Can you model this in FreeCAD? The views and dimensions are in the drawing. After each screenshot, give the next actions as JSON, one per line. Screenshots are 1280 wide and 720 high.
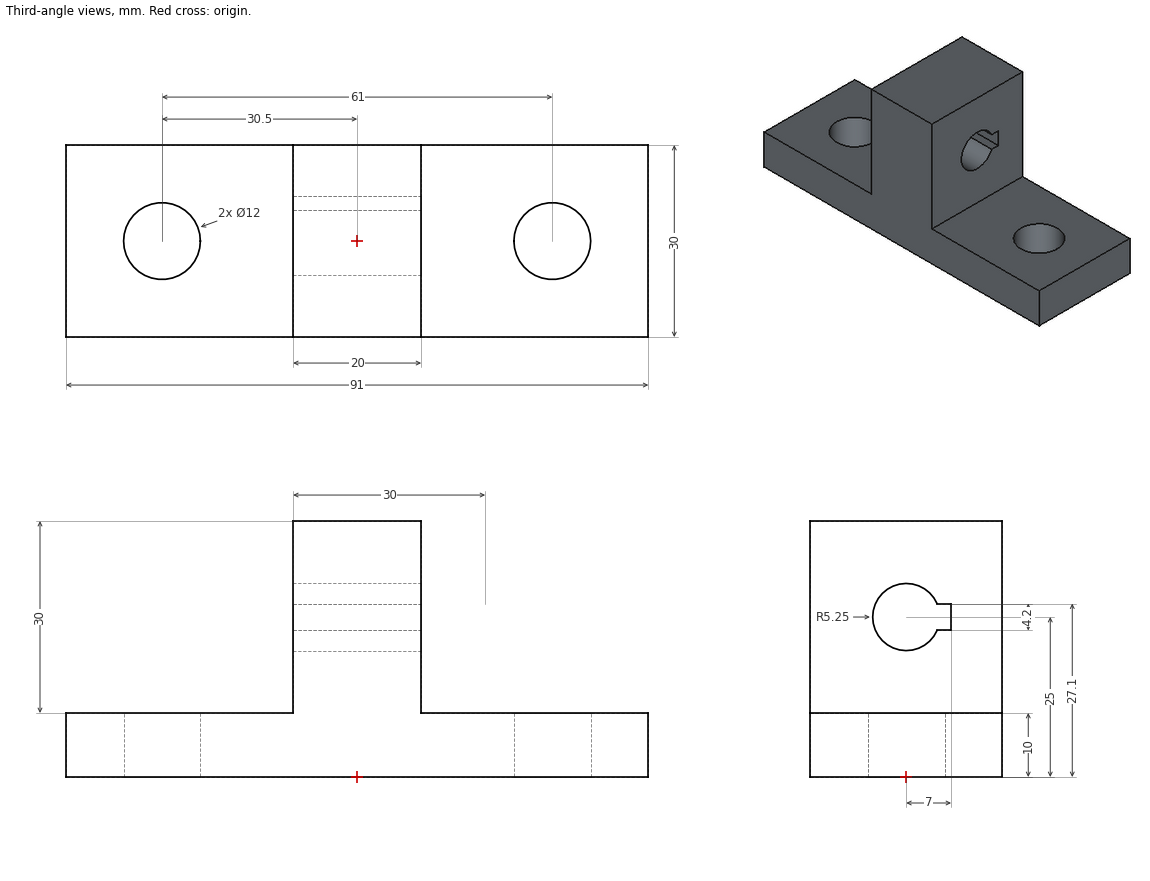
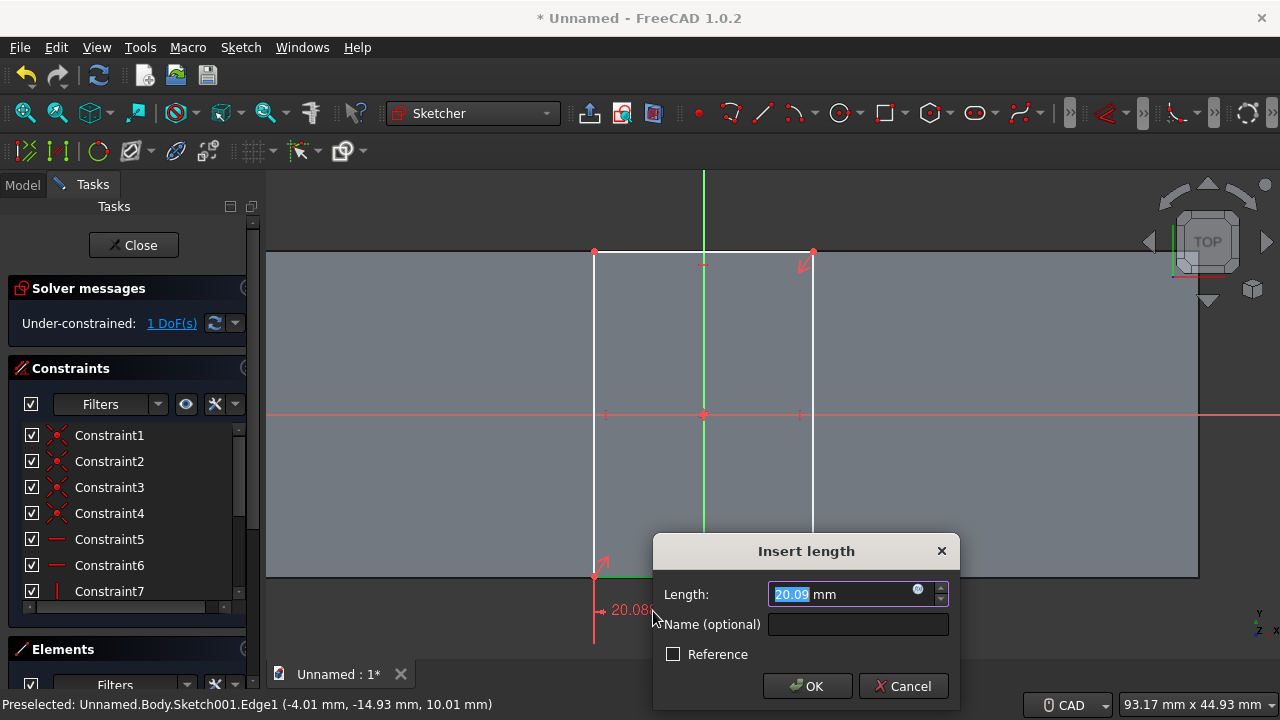
{"action": "type", "text": "20"}
{"action": "key", "text": "Return"}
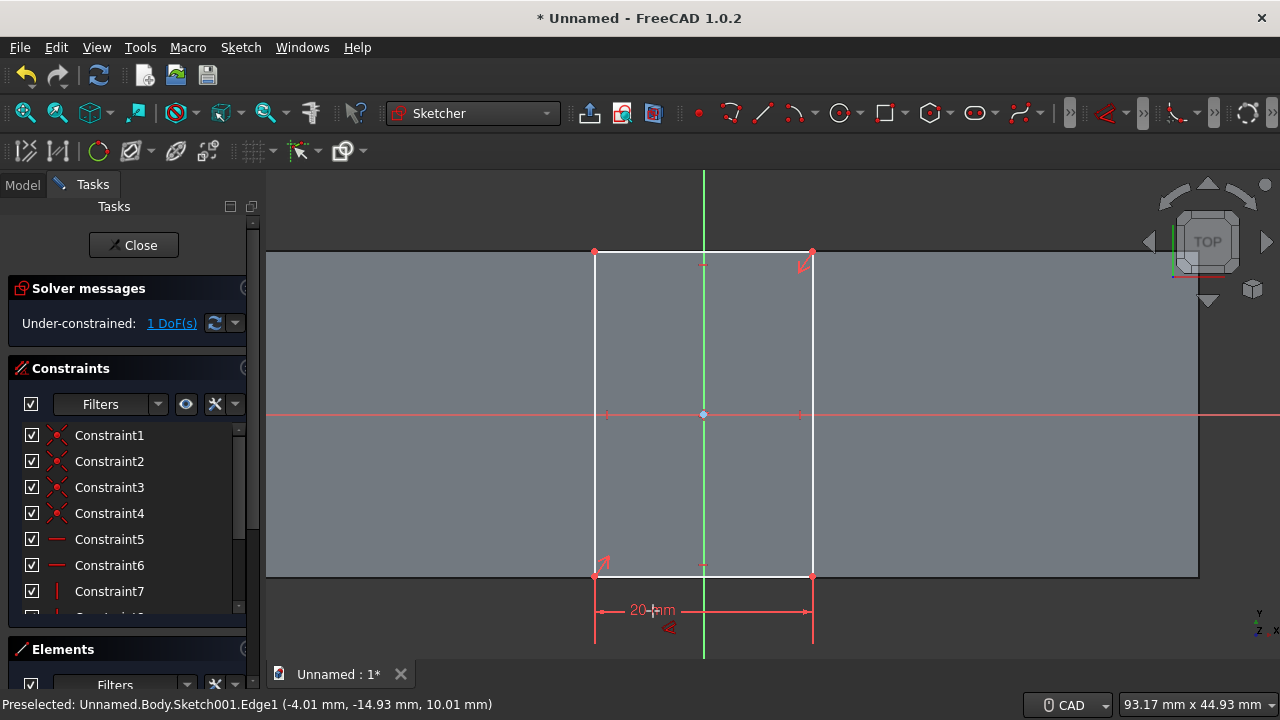
{"action": "left_click", "coordinate": [813, 480]}
{"action": "left_click", "coordinate": [847, 340]}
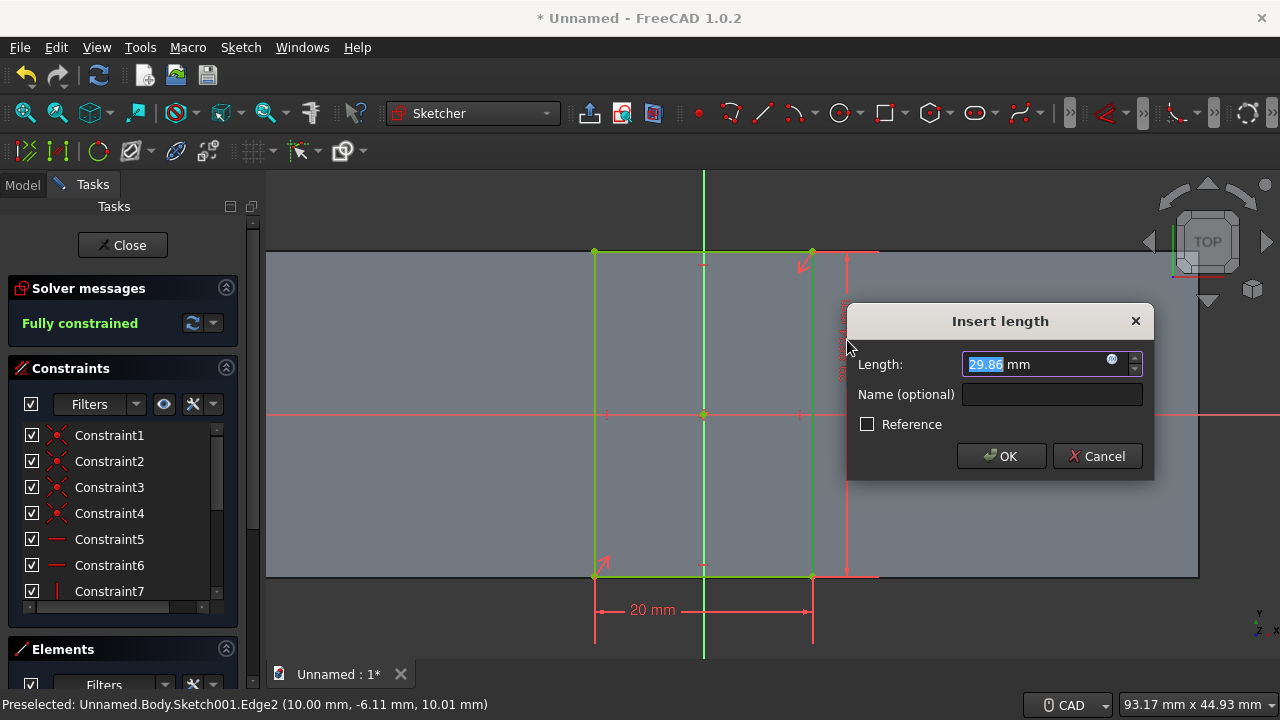
{"action": "type", "text": "30"}
{"action": "key", "text": "Return"}
{"action": "key", "text": "Escape"}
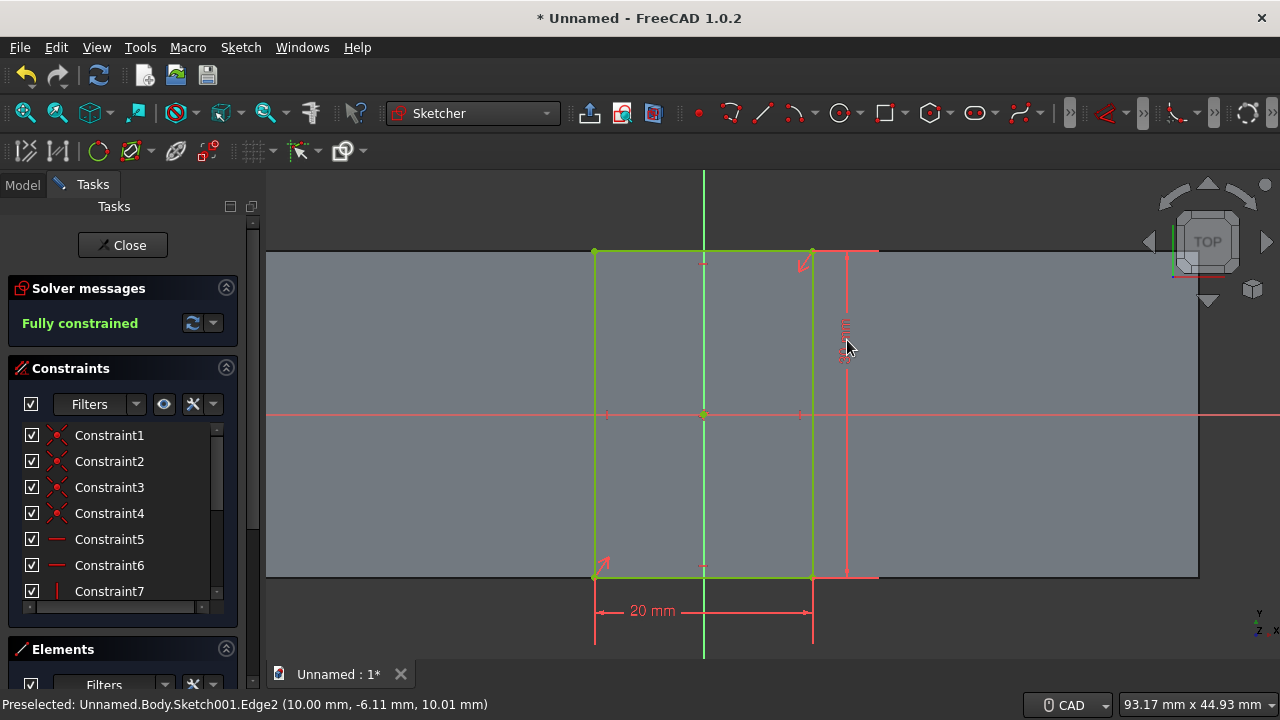
{"action": "left_click", "coordinate": [123, 245]}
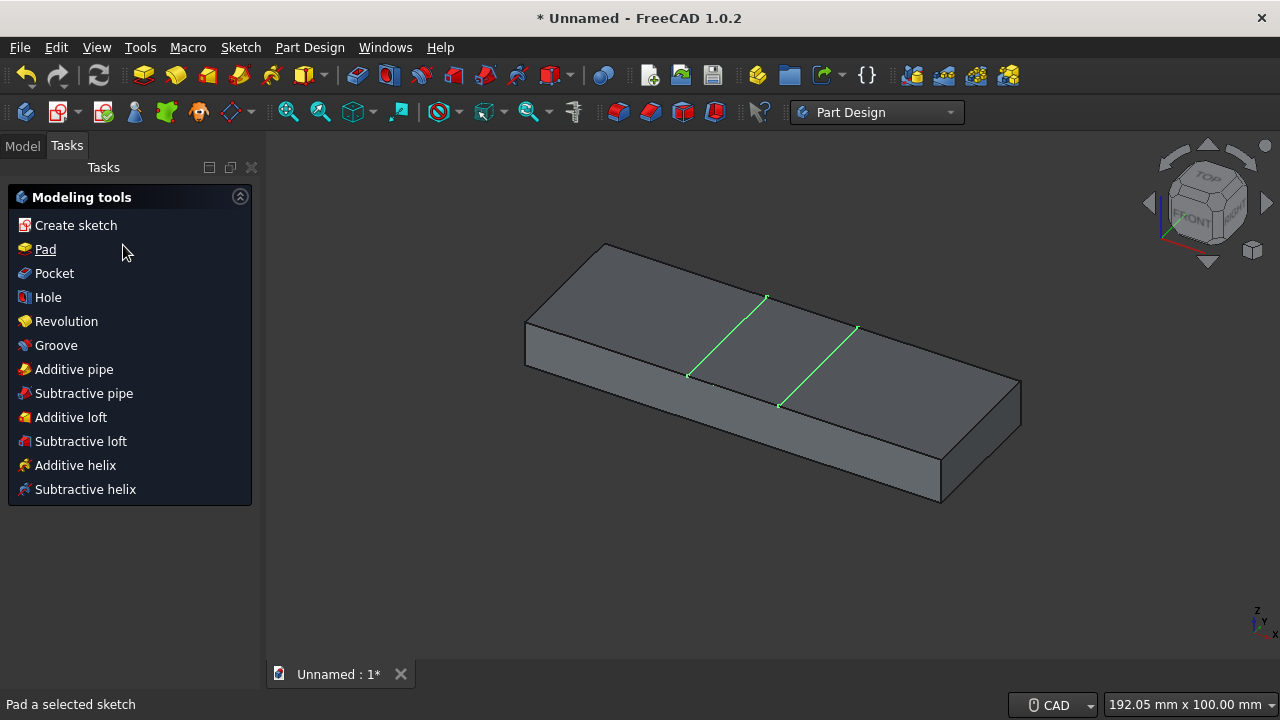
{"action": "left_click", "coordinate": [144, 76]}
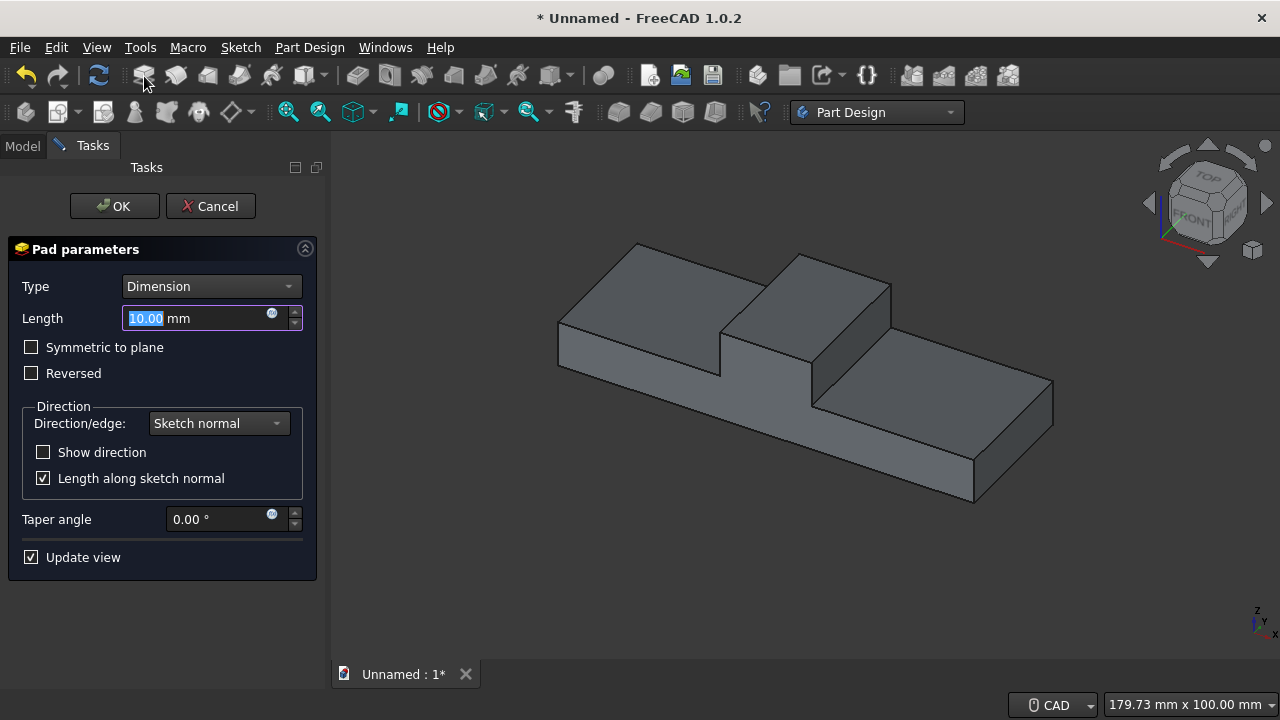
{"action": "type", "text": "30"}
{"action": "key", "text": "Tab"}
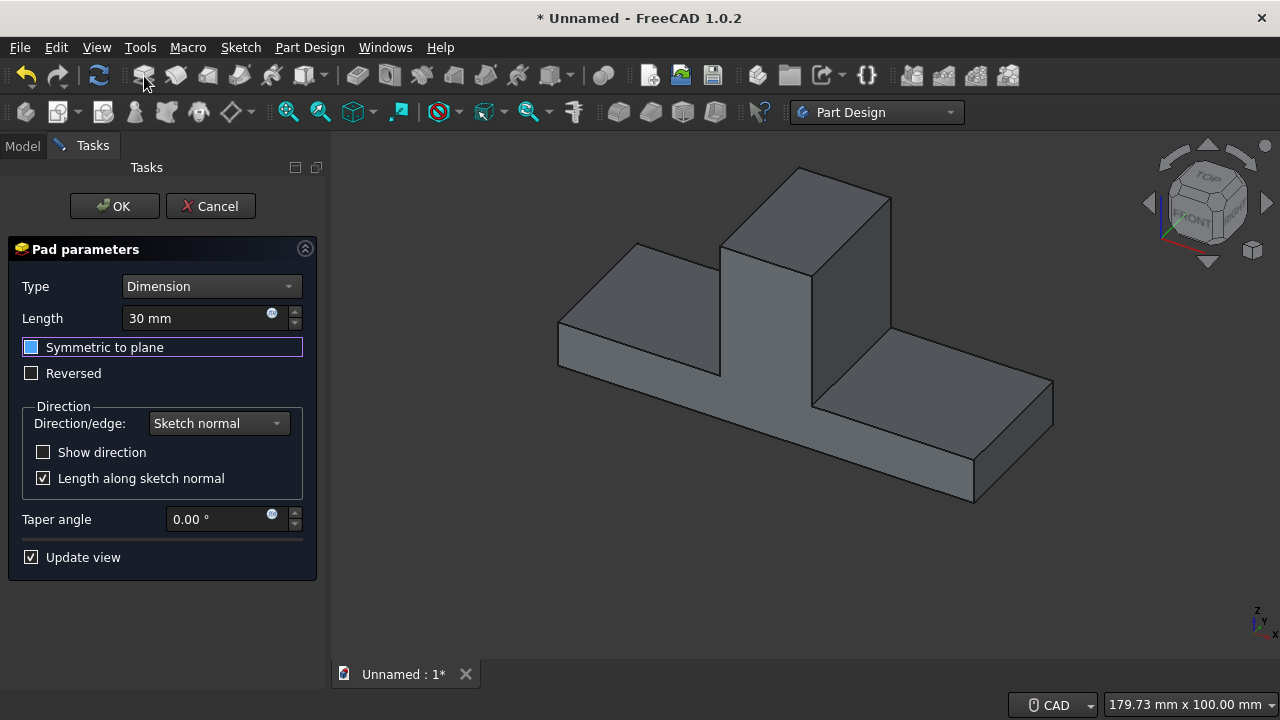
{"action": "left_click", "coordinate": [115, 206]}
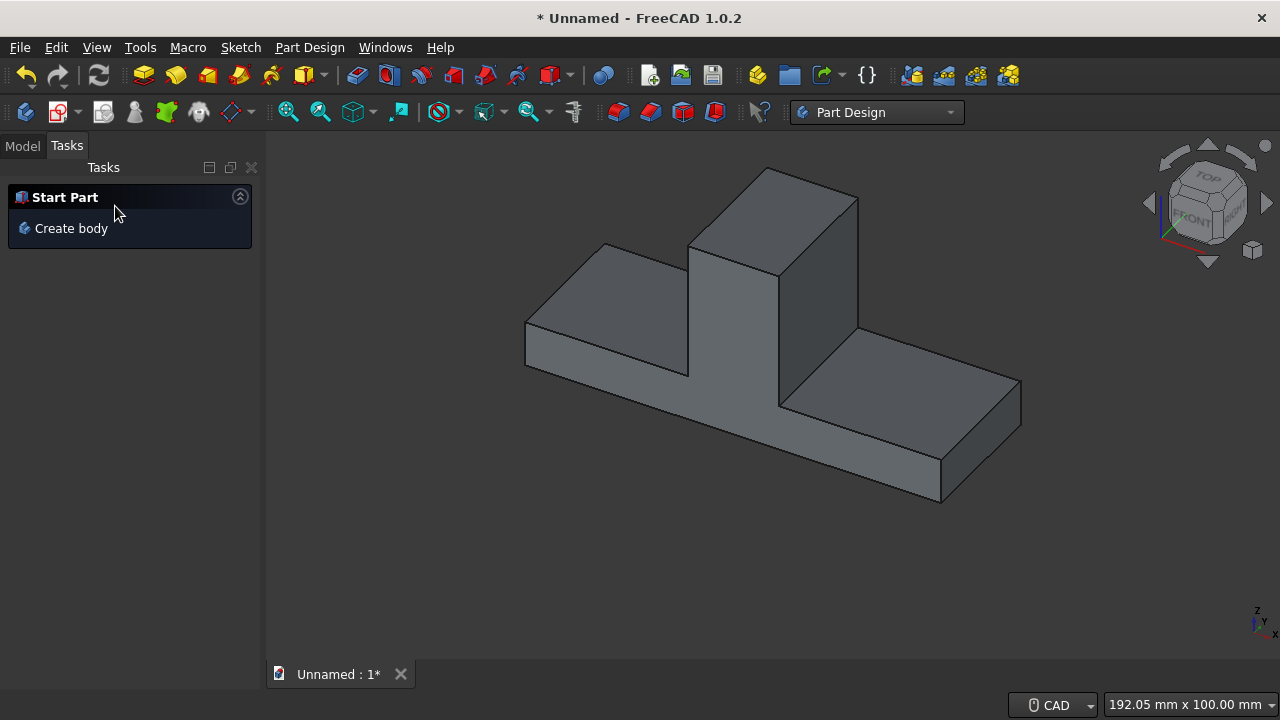
{"action": "key", "text": "v f"}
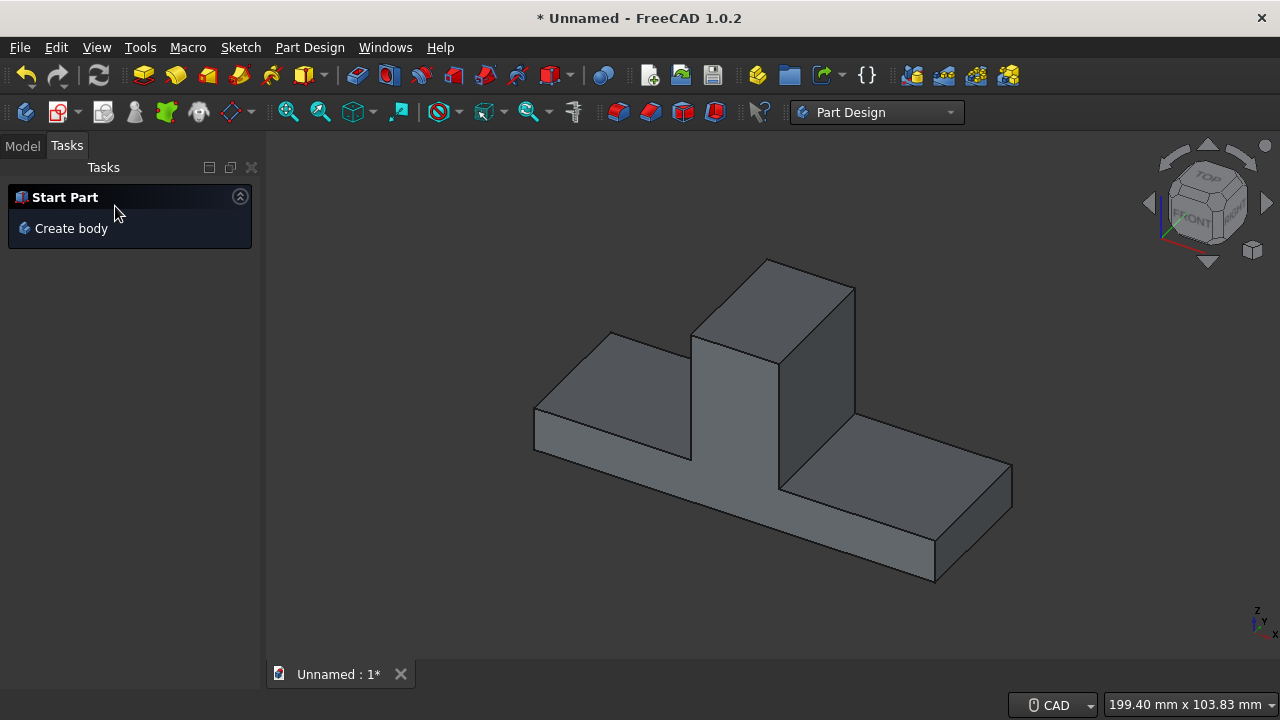
{"action": "key", "text": "6"}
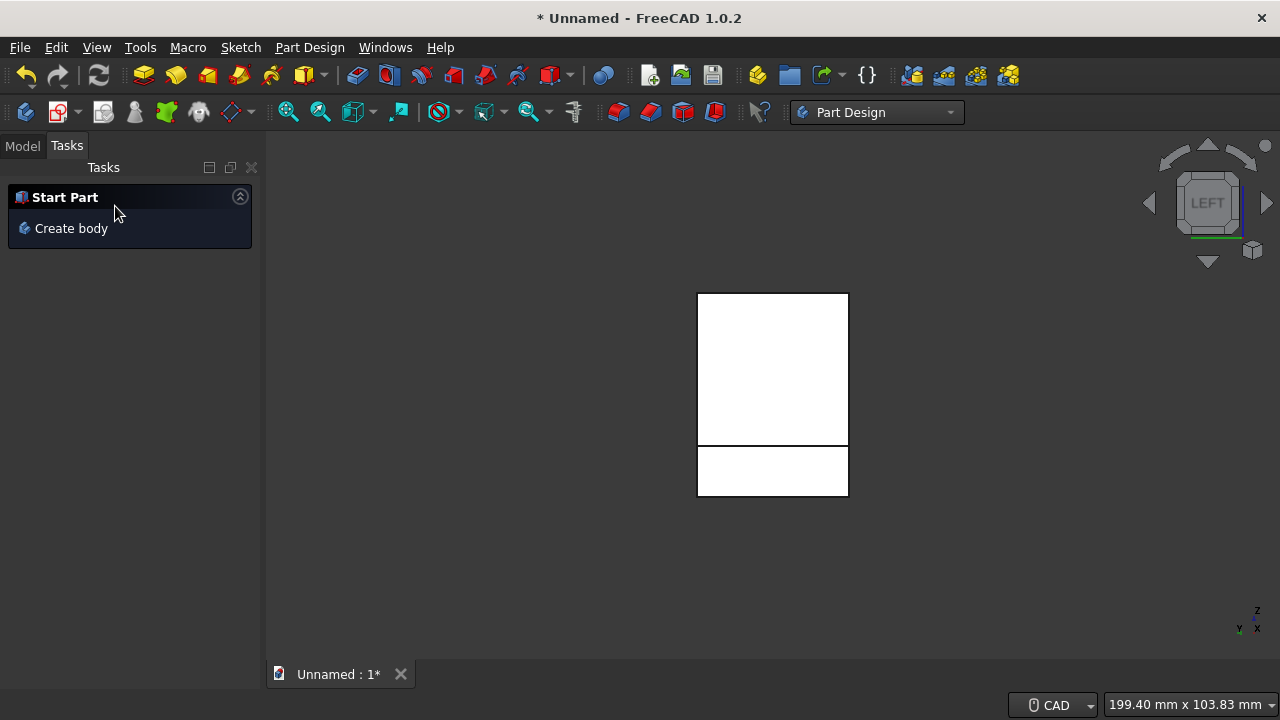
{"action": "left_click", "coordinate": [290, 112]}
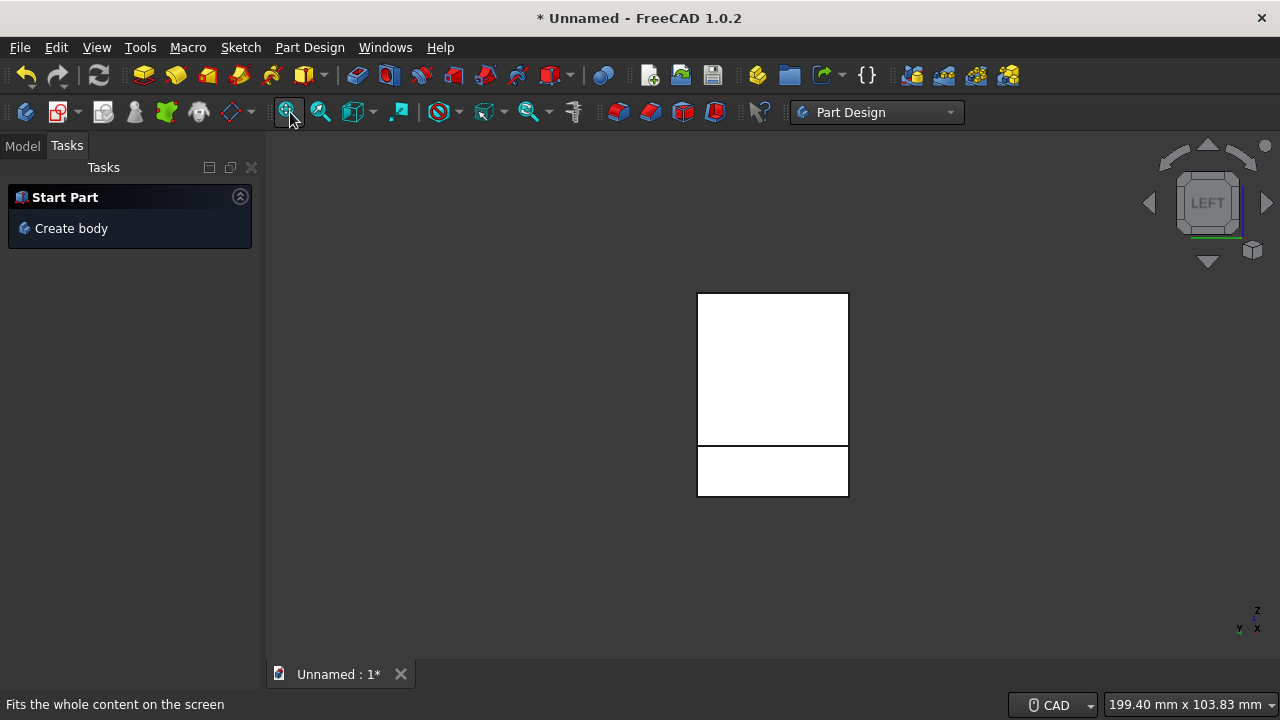
{"action": "left_click", "coordinate": [773, 369]}